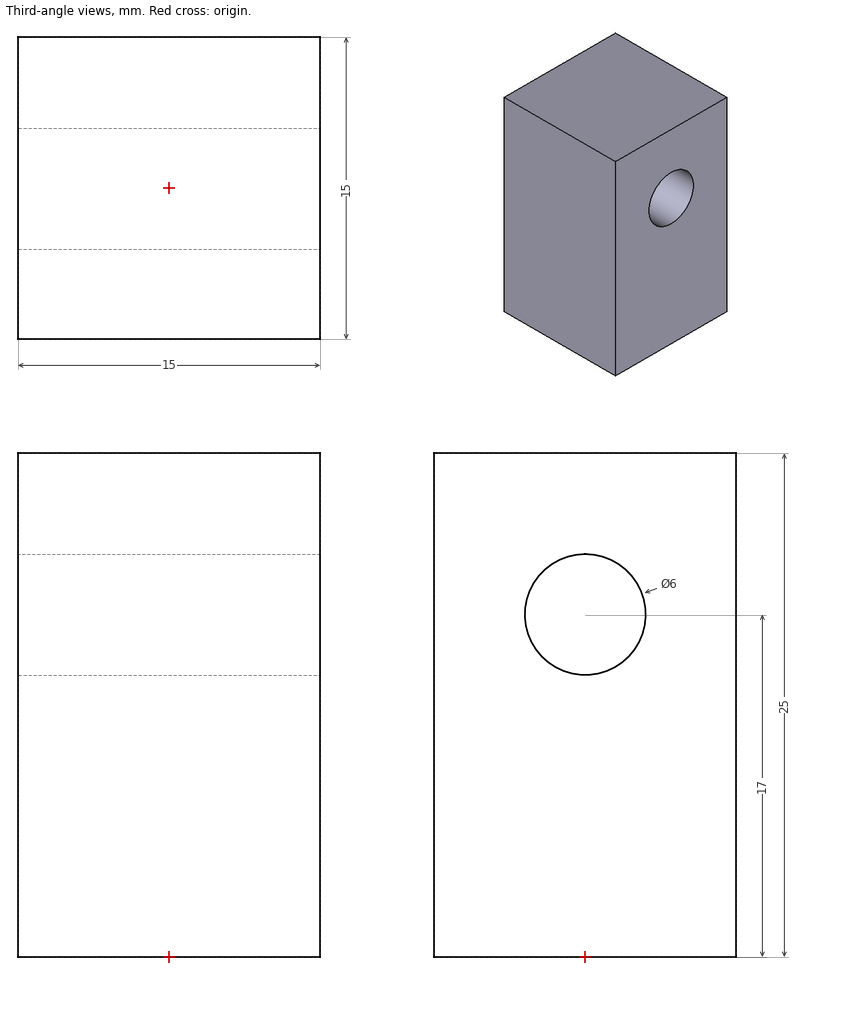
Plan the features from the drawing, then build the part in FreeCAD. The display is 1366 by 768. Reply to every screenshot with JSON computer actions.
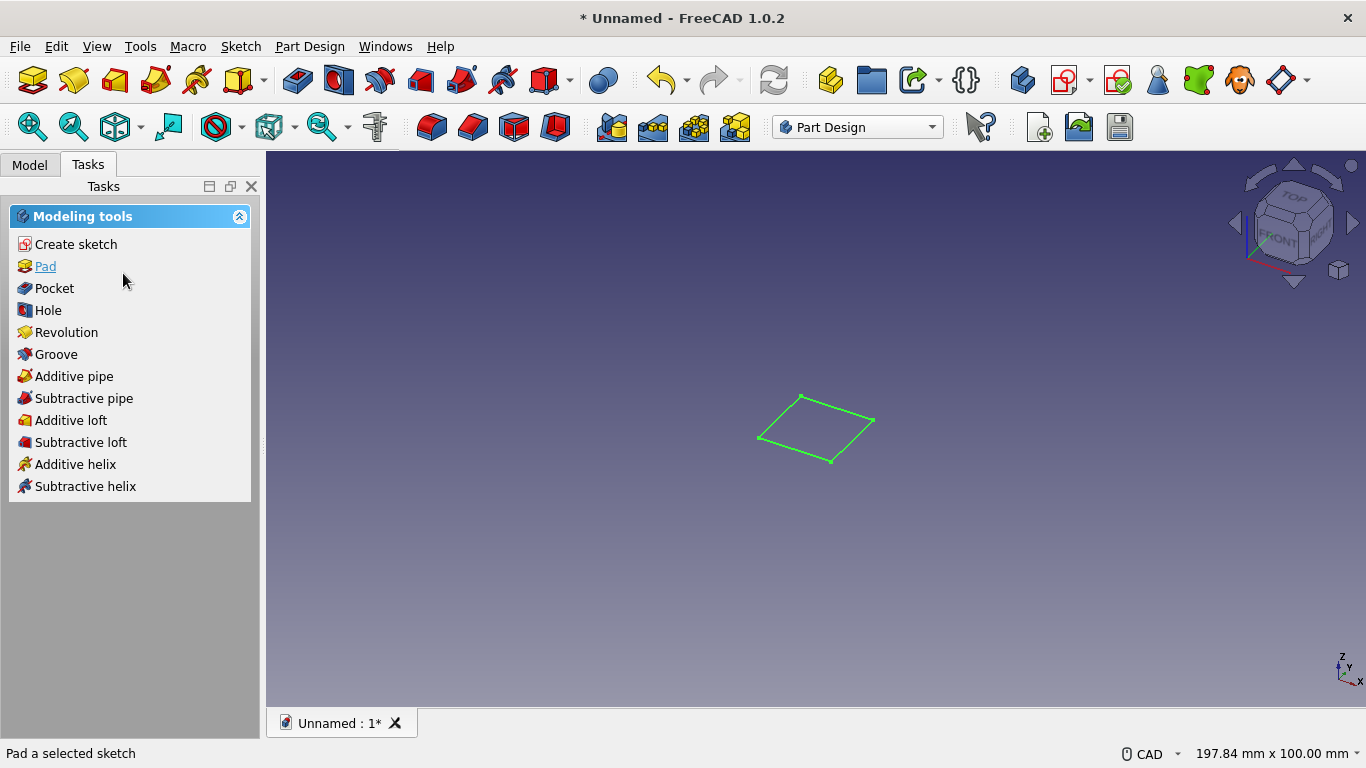
{"action": "left_click", "coordinate": [33, 80]}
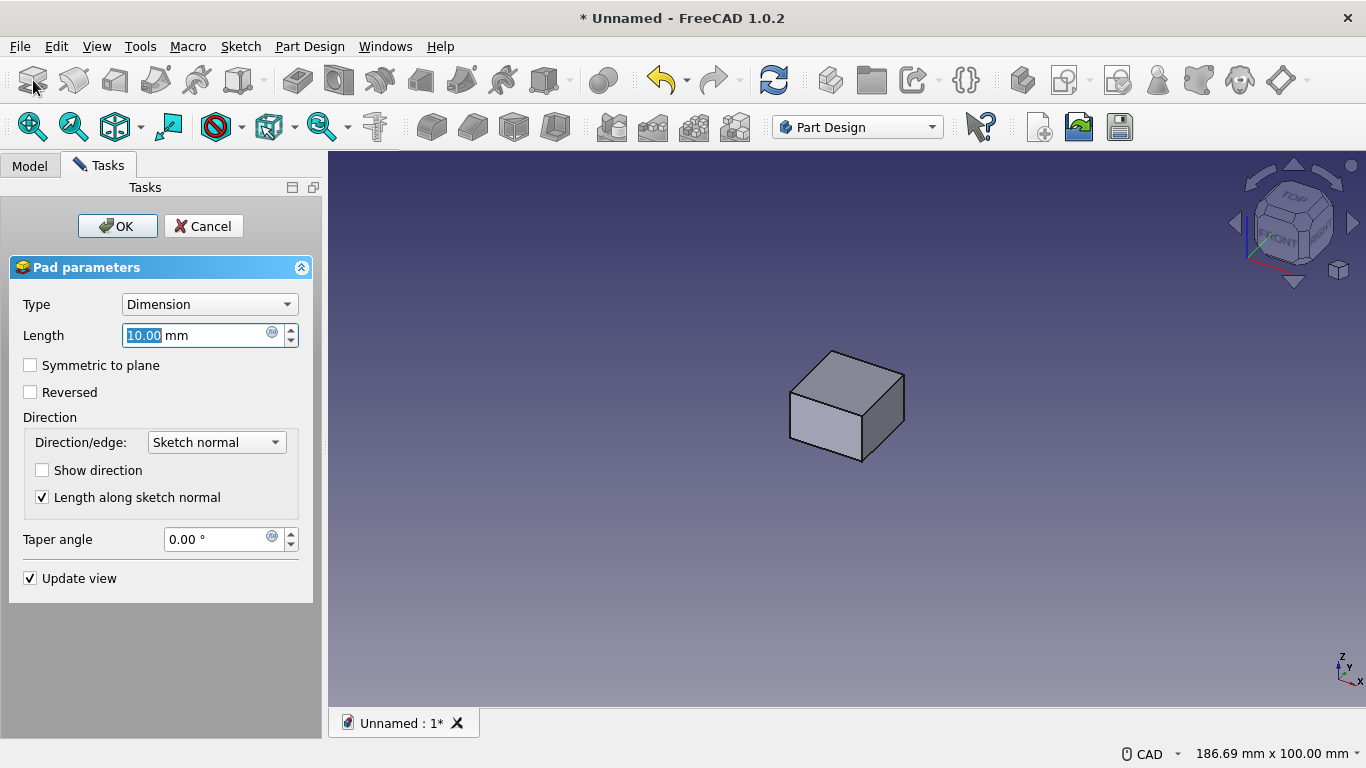
{"action": "type", "text": "25"}
{"action": "key", "text": "Tab"}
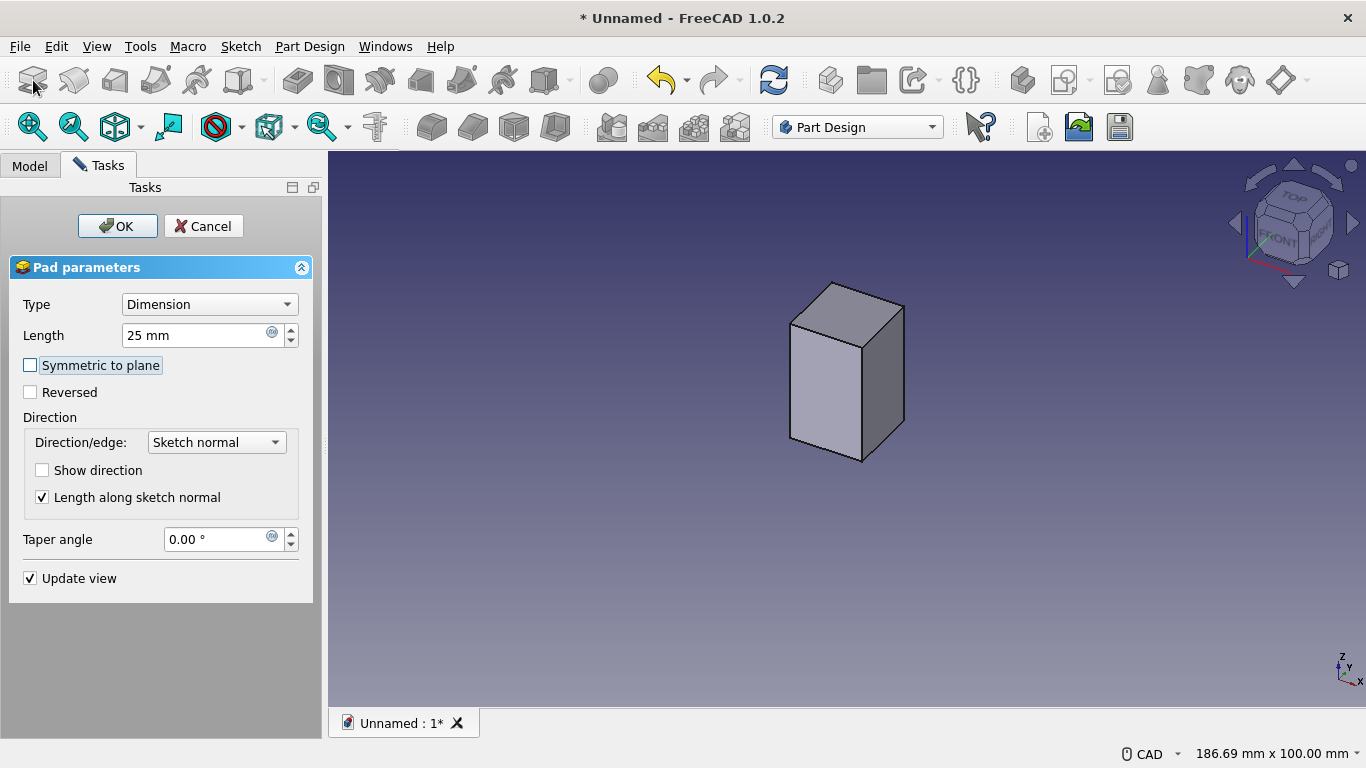
{"action": "left_click", "coordinate": [118, 226]}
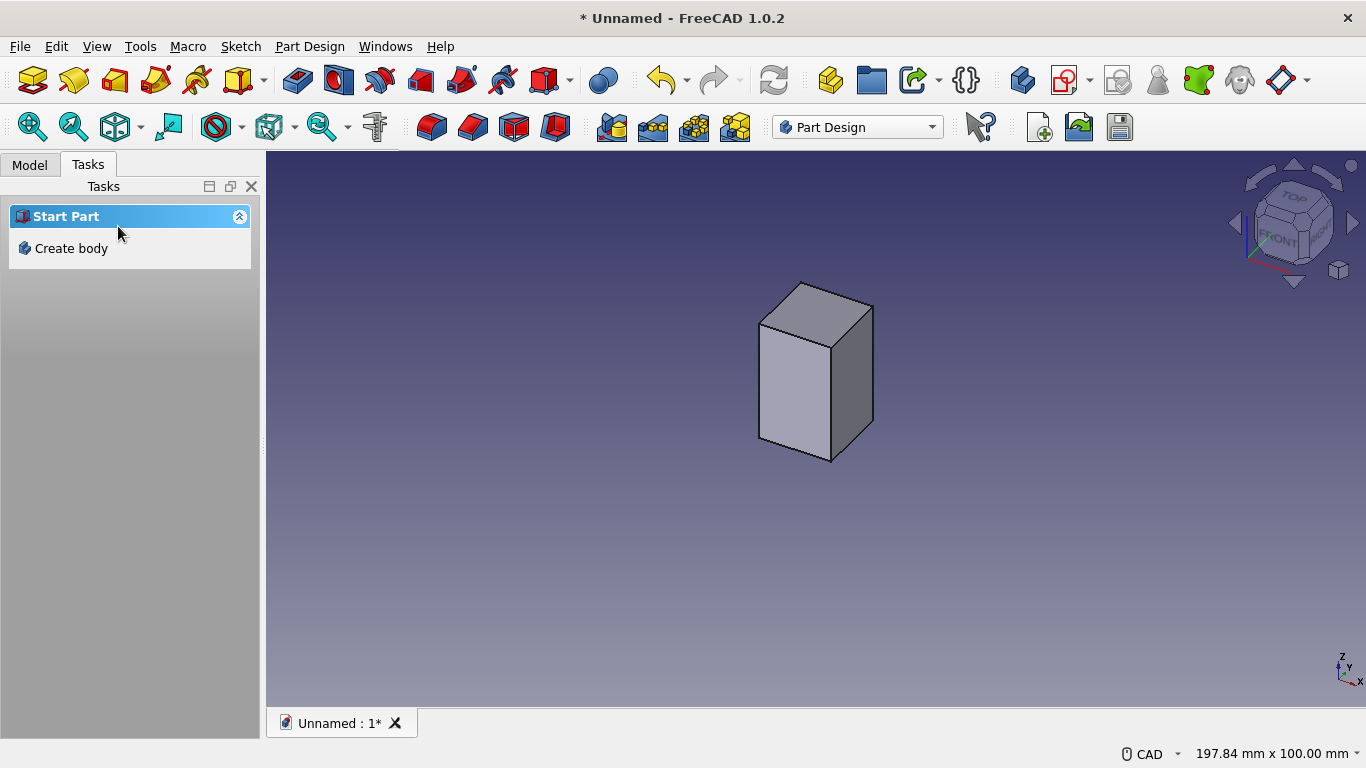
{"action": "key", "text": "v f"}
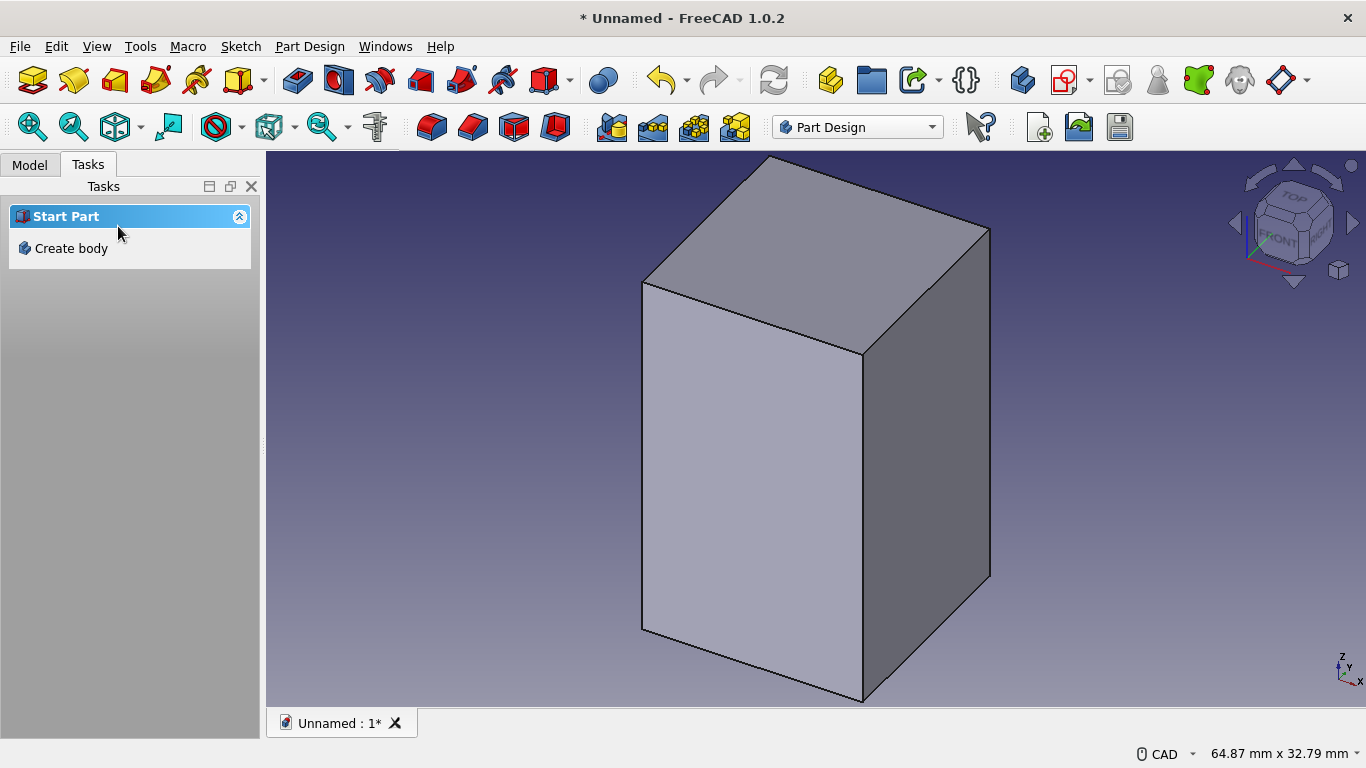
{"action": "key", "text": "6"}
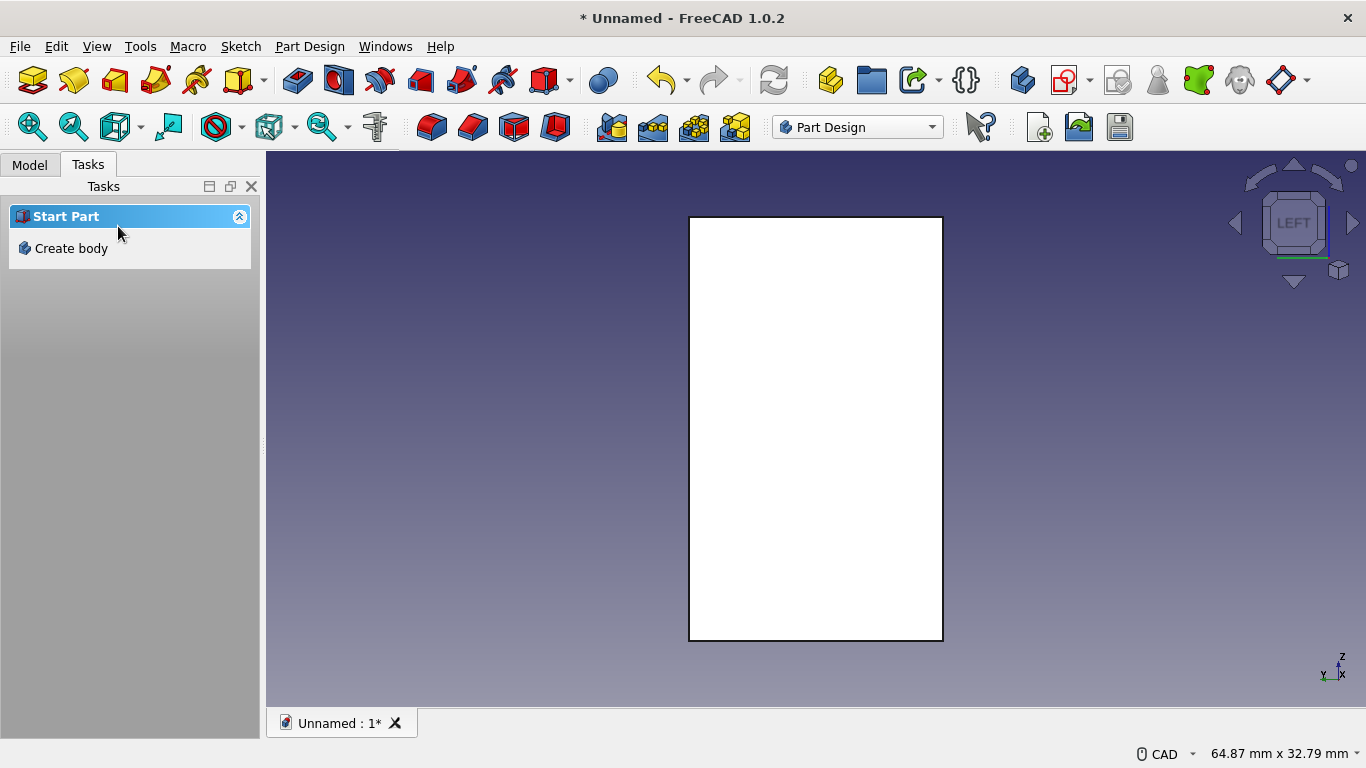
{"action": "left_click", "coordinate": [816, 367]}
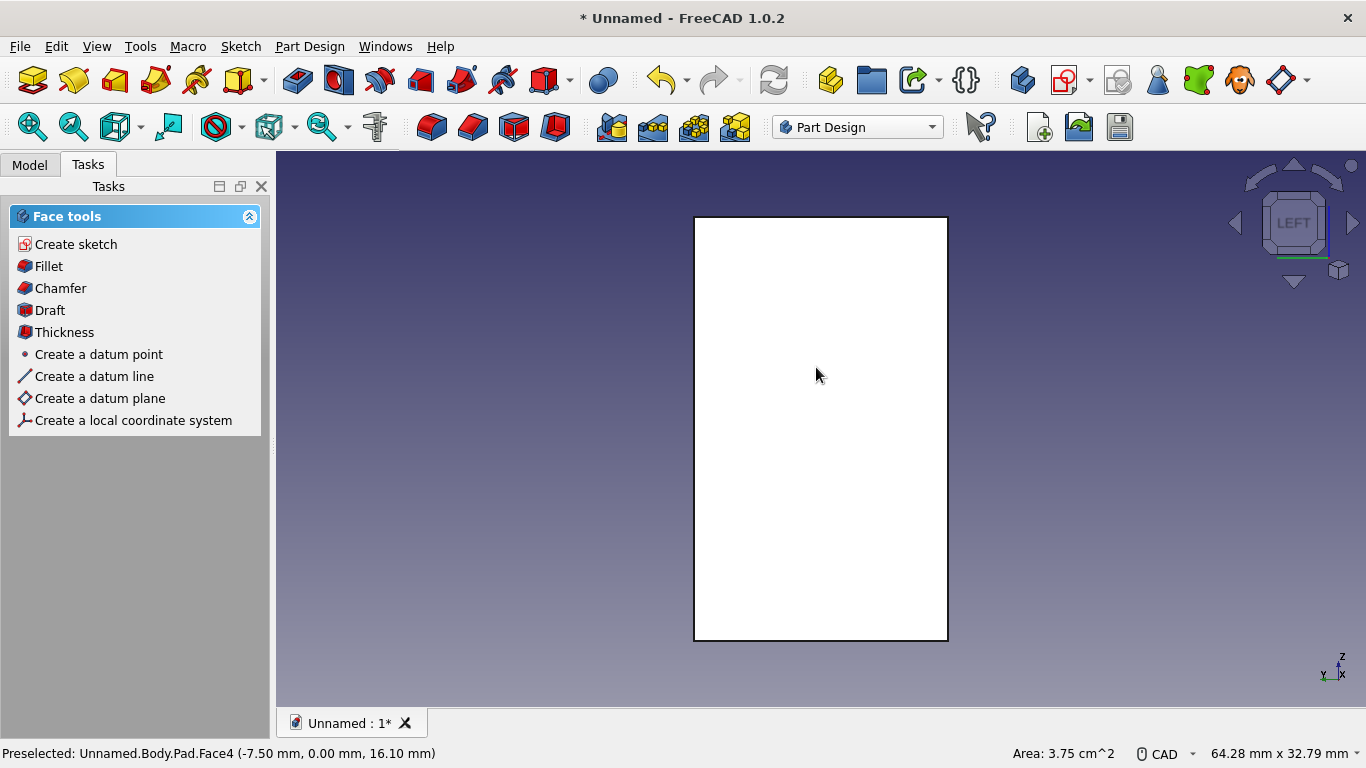
{"action": "left_click", "coordinate": [1064, 80]}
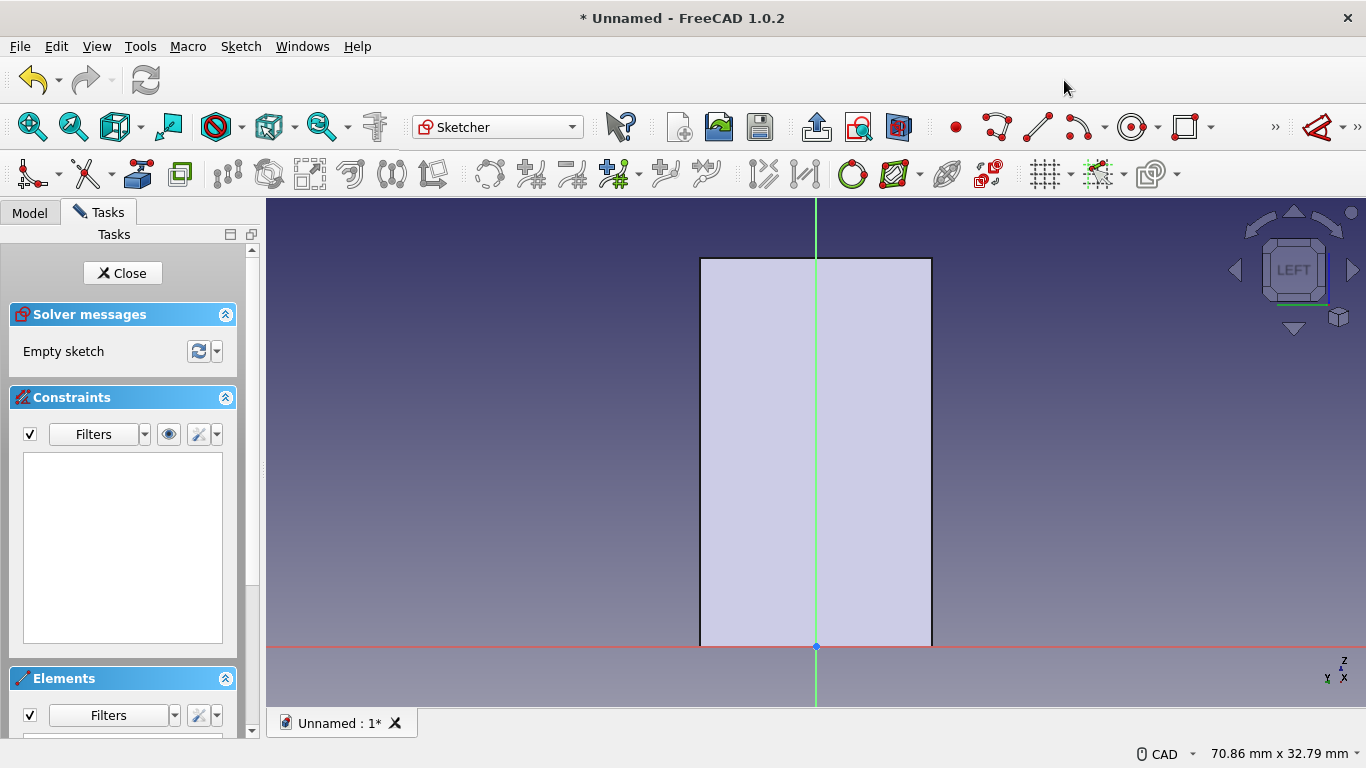
{"action": "scroll", "coordinate": [846, 353], "scroll_direction": "up", "scroll_amount": 6}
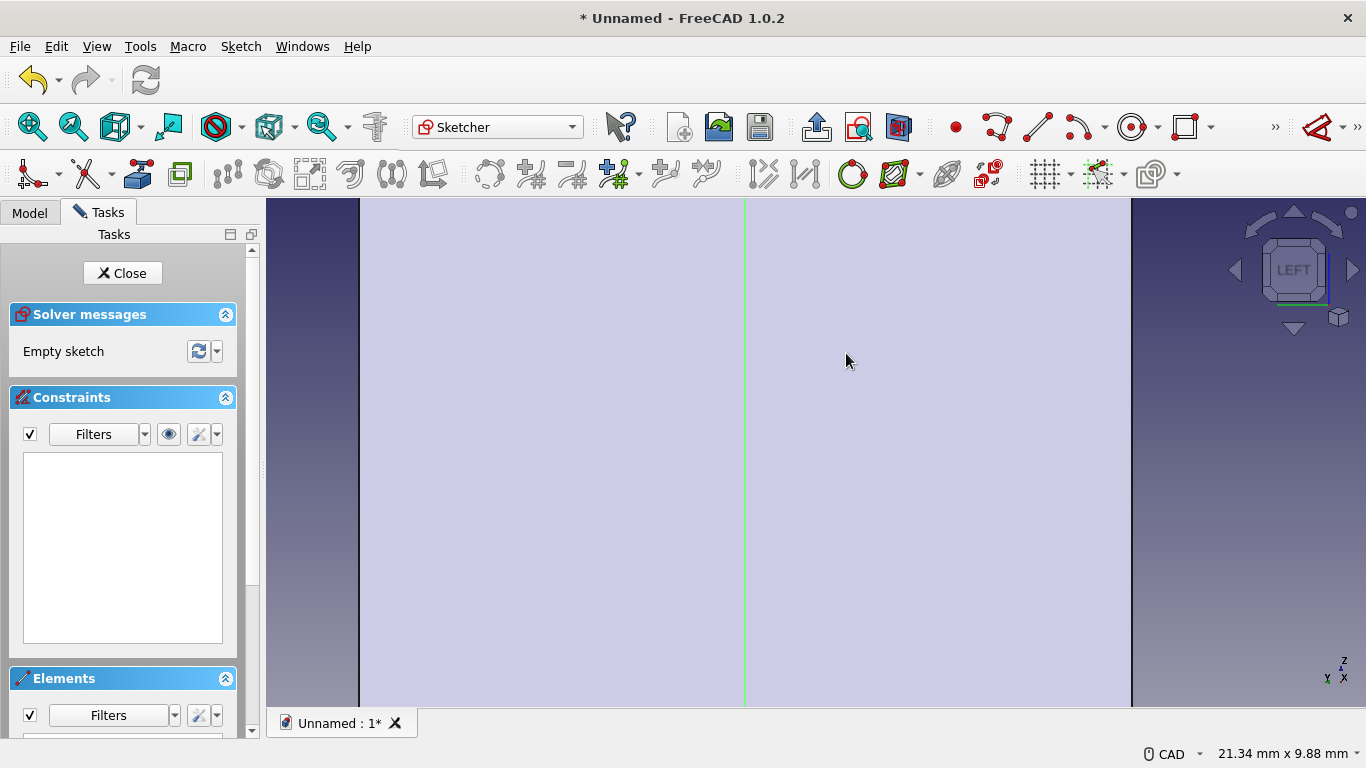
{"action": "key", "text": "g c"}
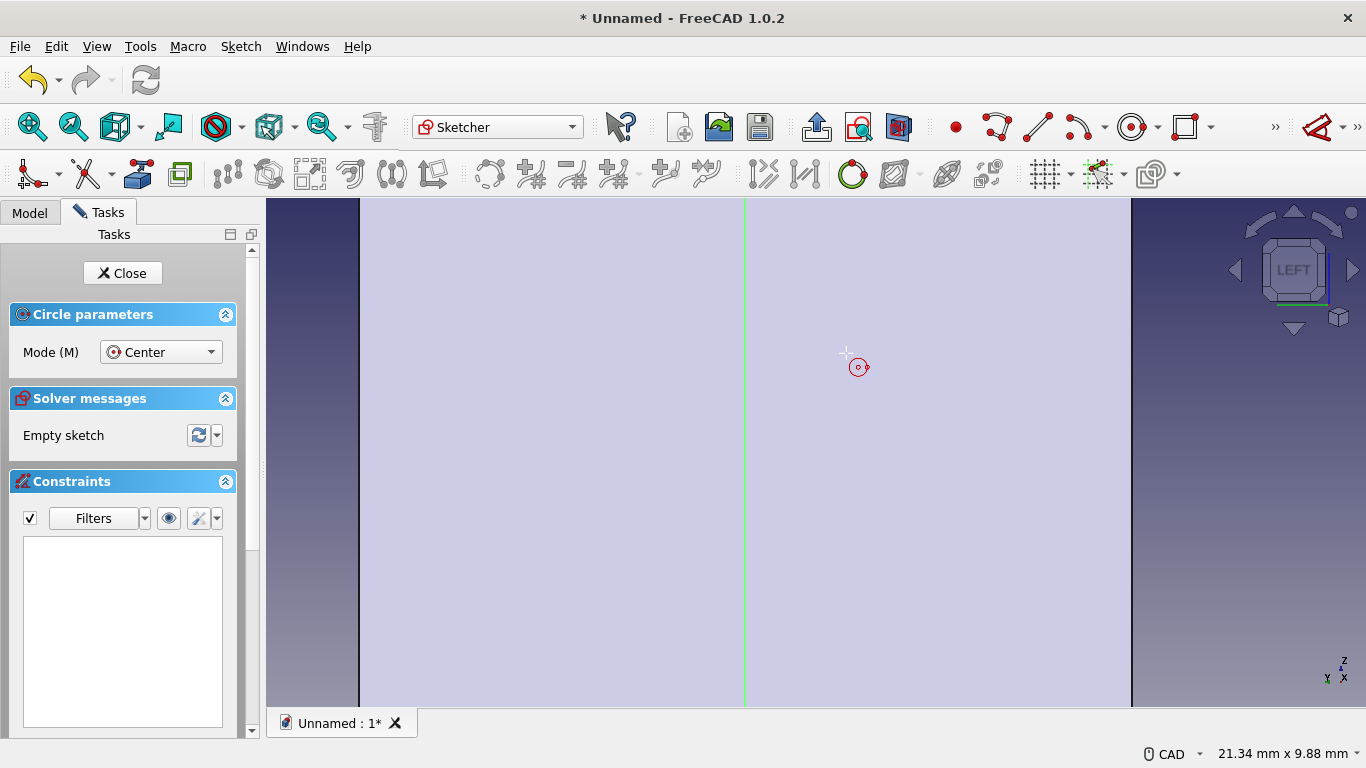
{"action": "left_click", "coordinate": [745, 451]}
{"action": "mouse_move", "coordinate": [855, 341]}